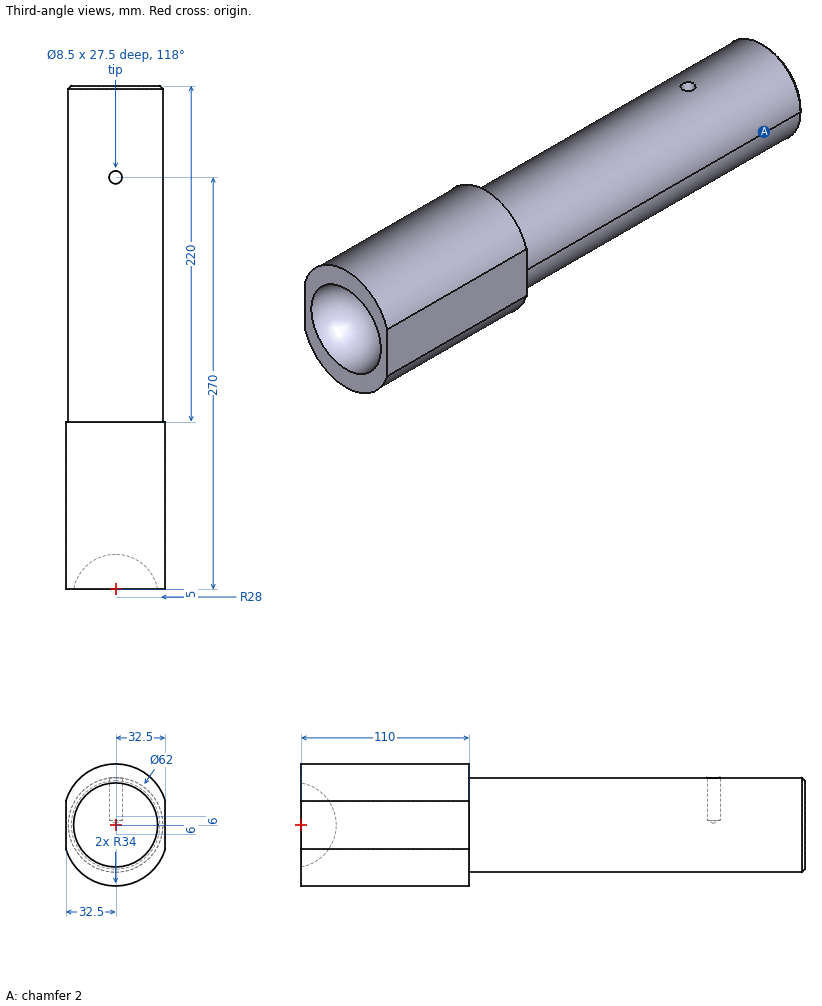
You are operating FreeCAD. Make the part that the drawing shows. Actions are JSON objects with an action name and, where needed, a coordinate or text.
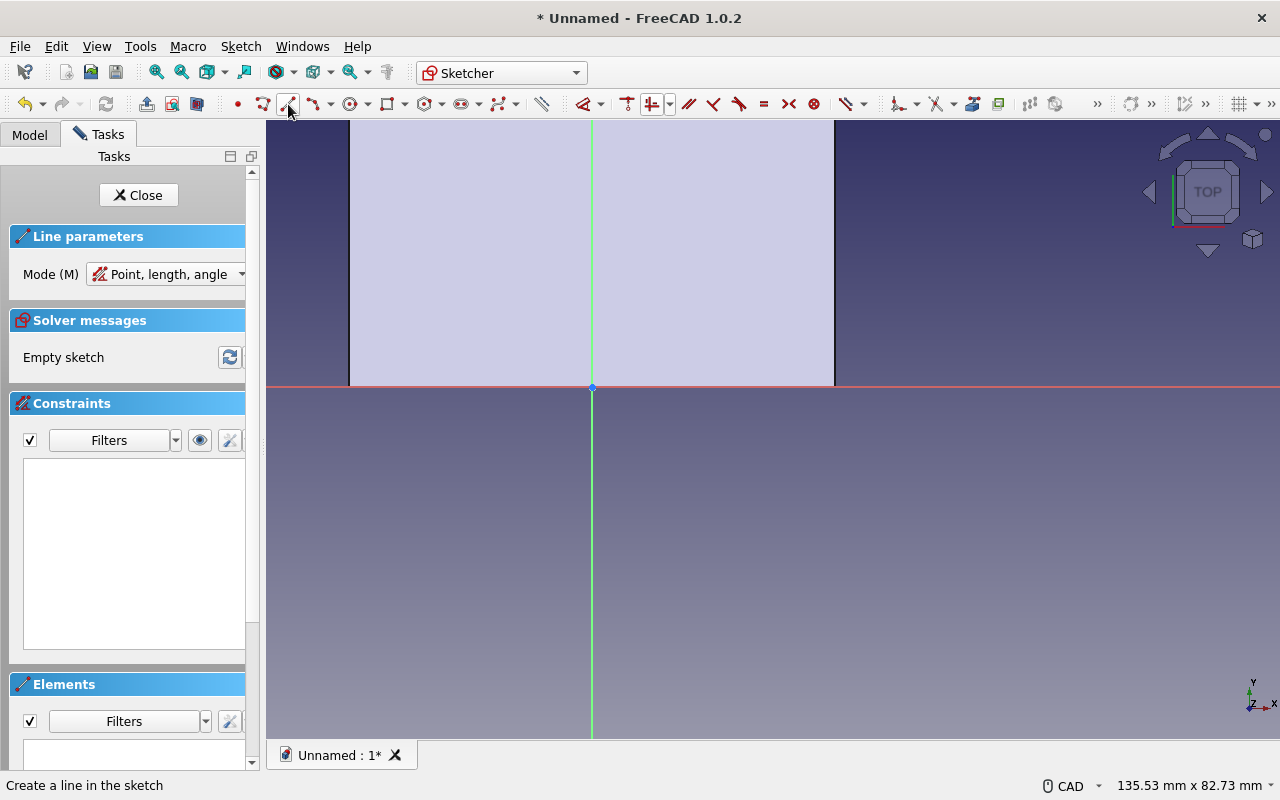
{"action": "left_click", "coordinate": [592, 215]}
{"action": "left_click", "coordinate": [601, 634]}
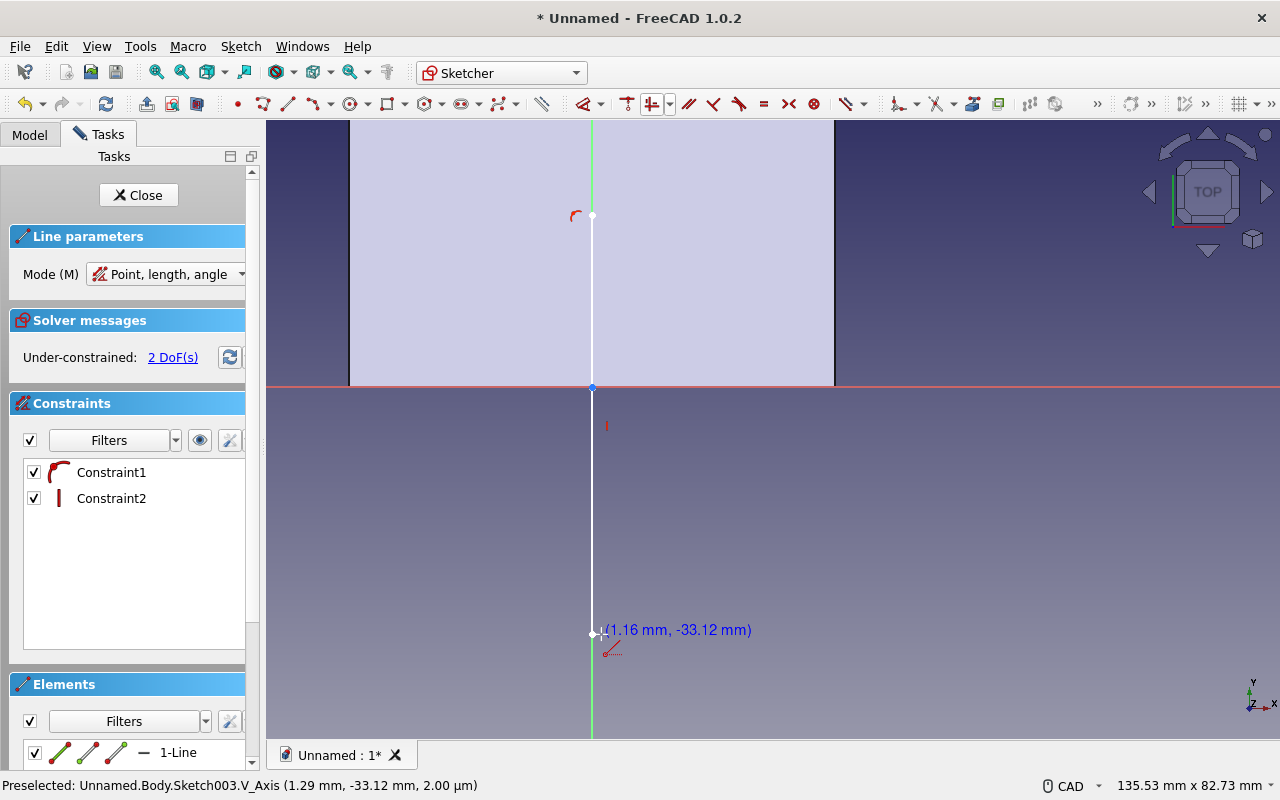
{"action": "key", "text": "g 3 a"}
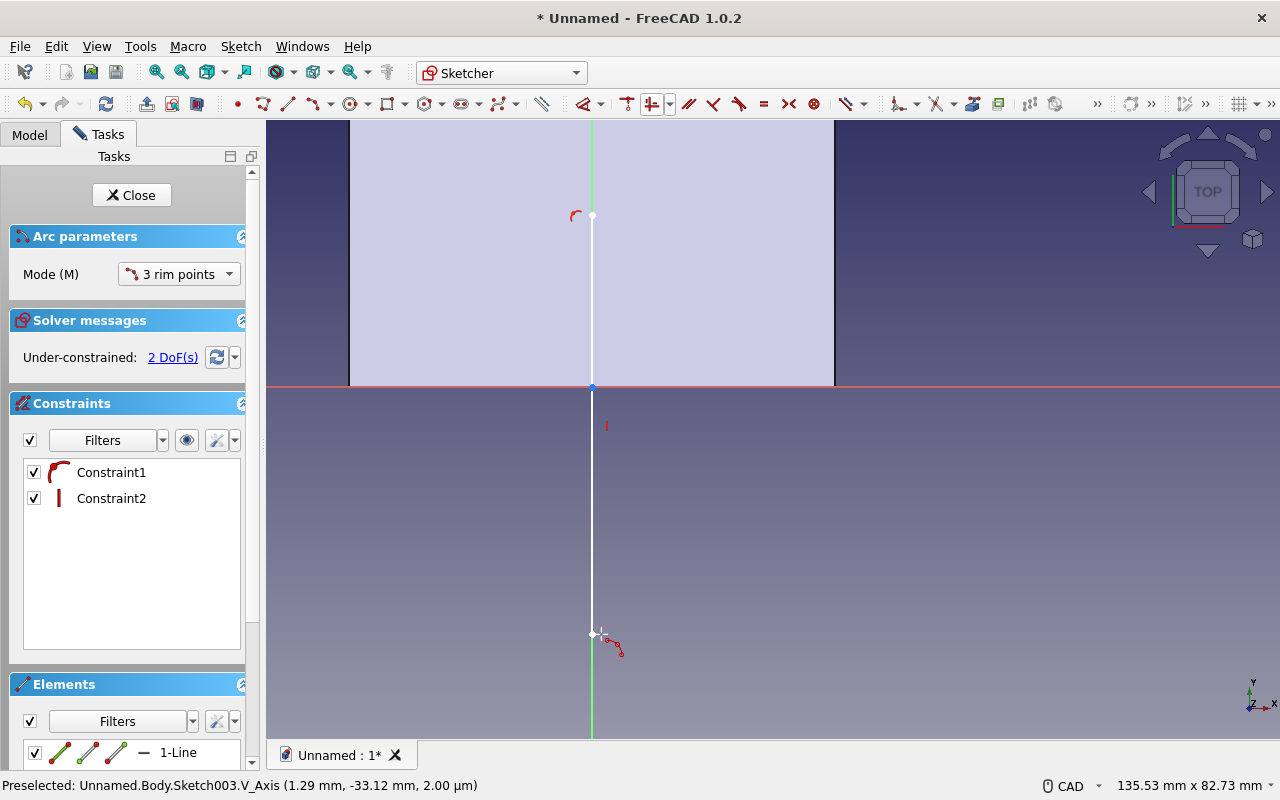
{"action": "left_click", "coordinate": [592, 635]}
{"action": "left_click", "coordinate": [592, 216]}
{"action": "left_click", "coordinate": [802, 425]}
{"action": "key", "text": "Escape"}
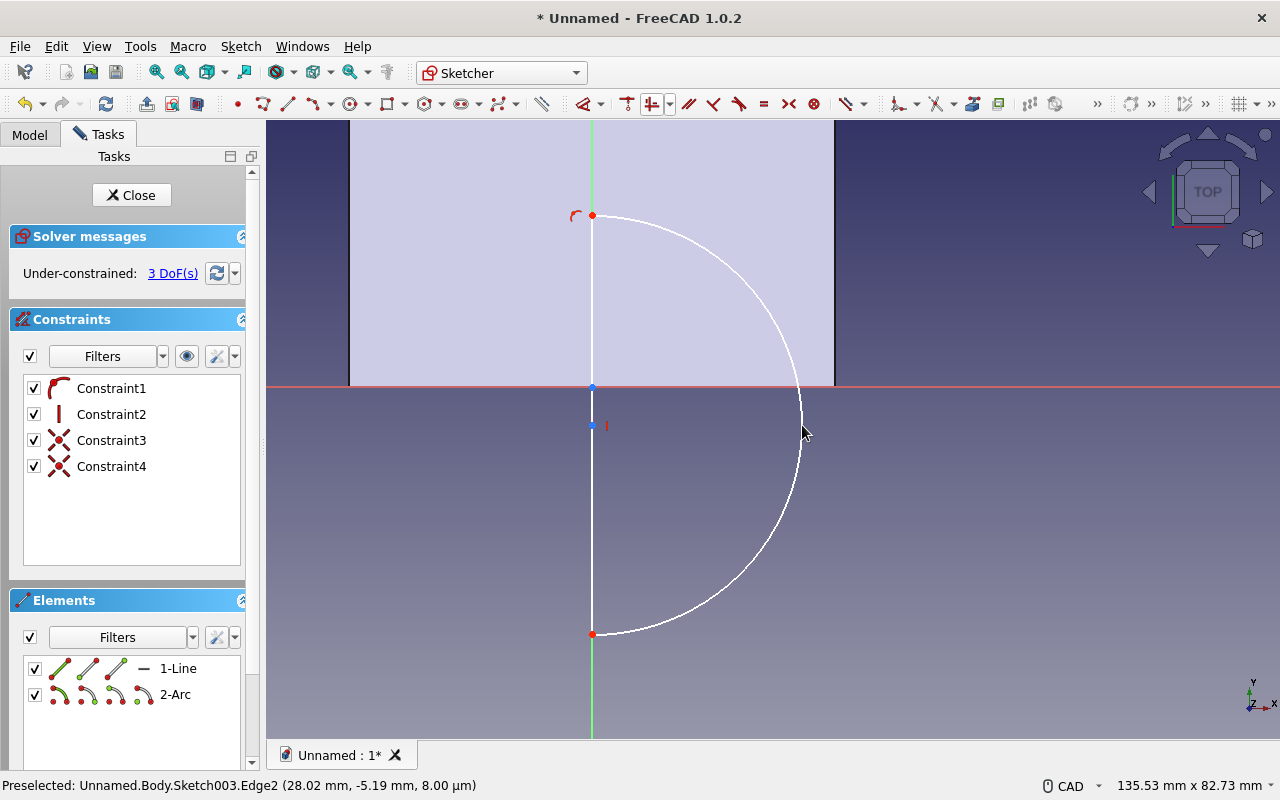
{"action": "left_click", "coordinate": [593, 425]}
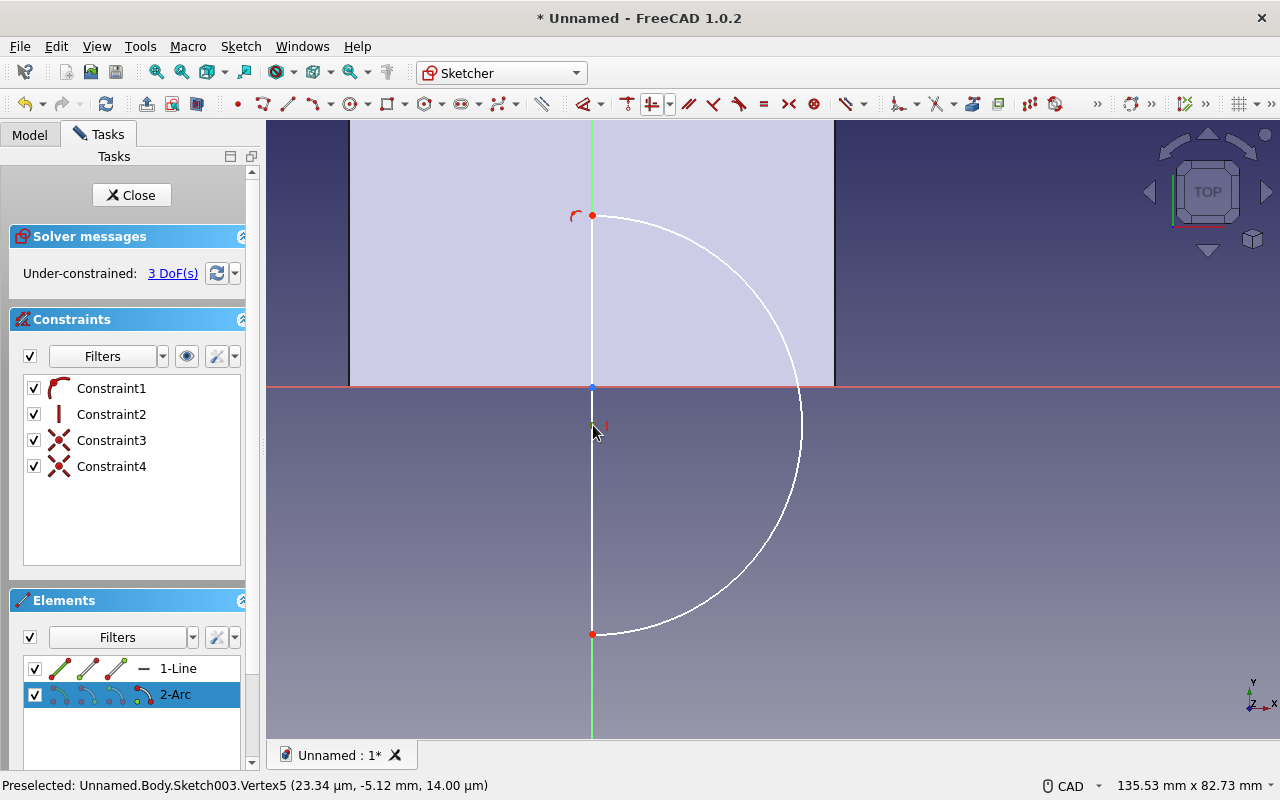
{"action": "left_click", "coordinate": [592, 671]}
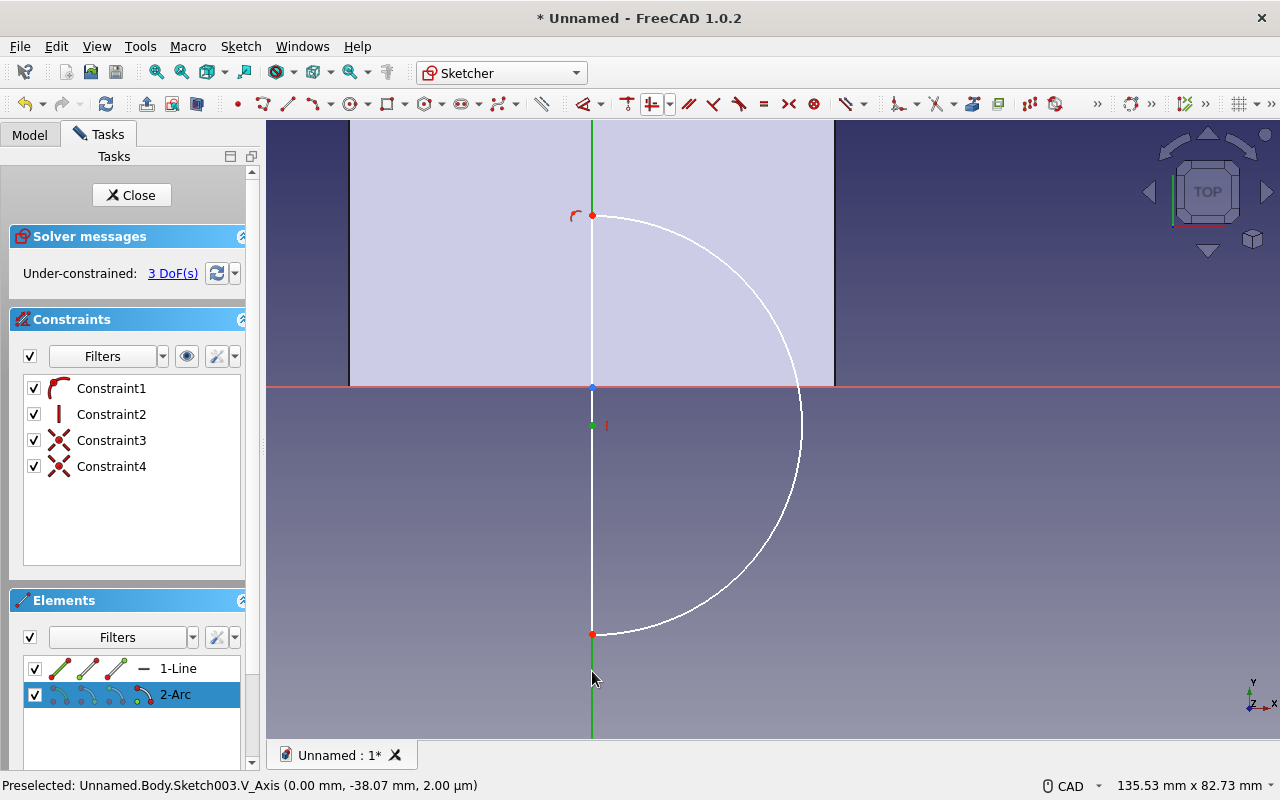
{"action": "left_click", "coordinate": [627, 104]}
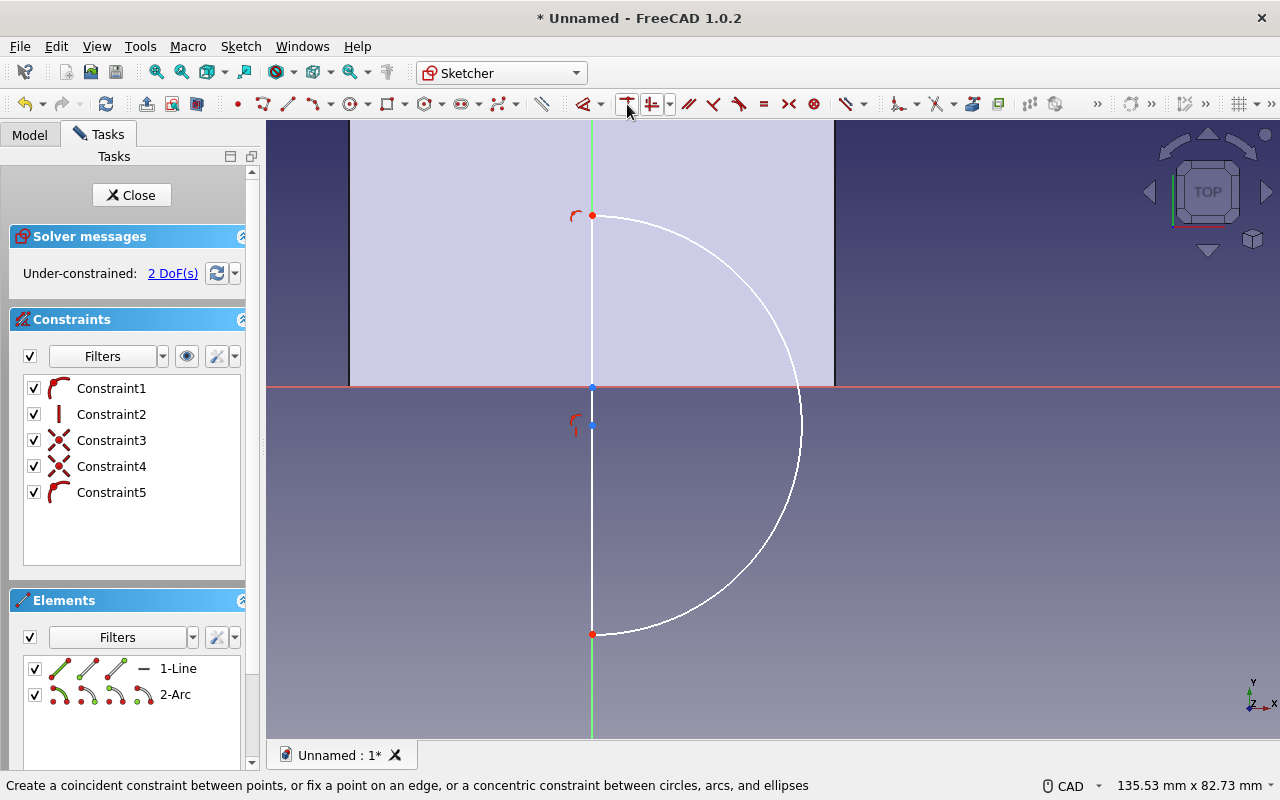
{"action": "left_click", "coordinate": [582, 104]}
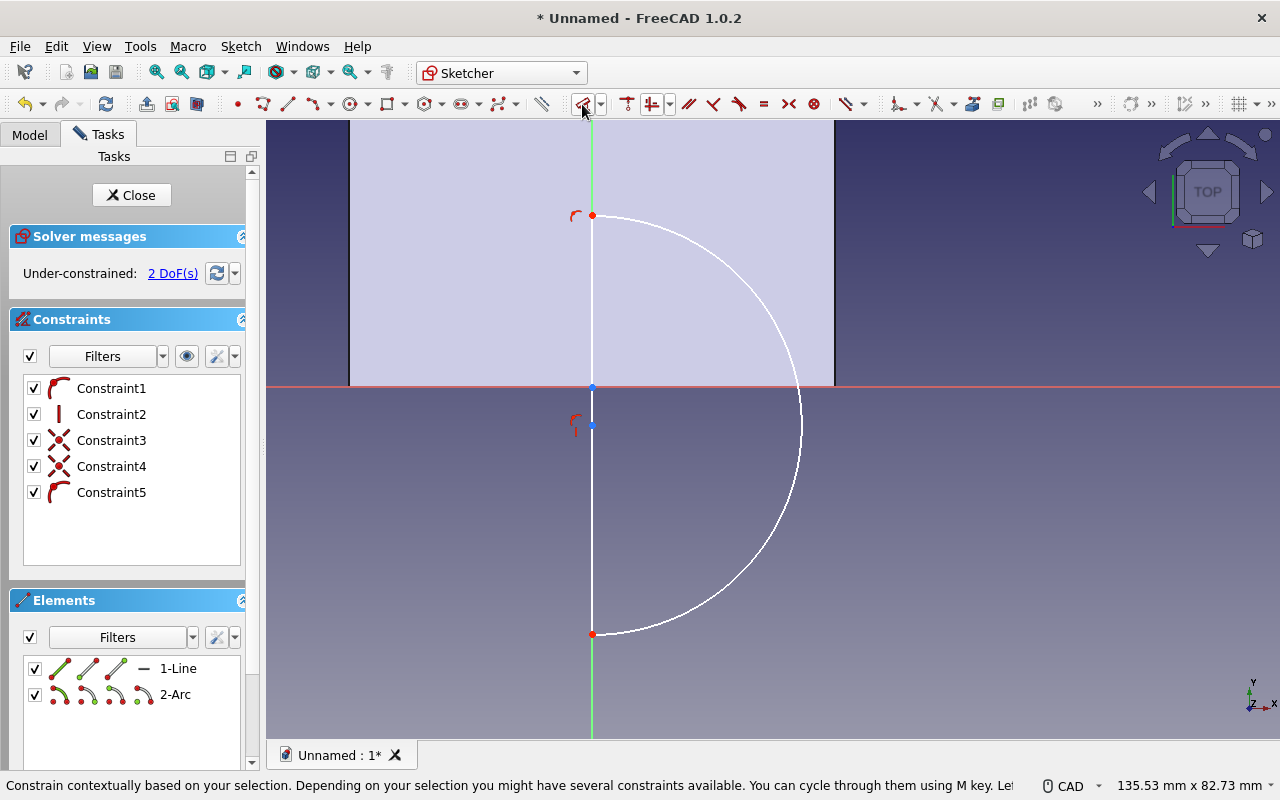
{"action": "left_click", "coordinate": [762, 549]}
{"action": "left_click", "coordinate": [788, 568]}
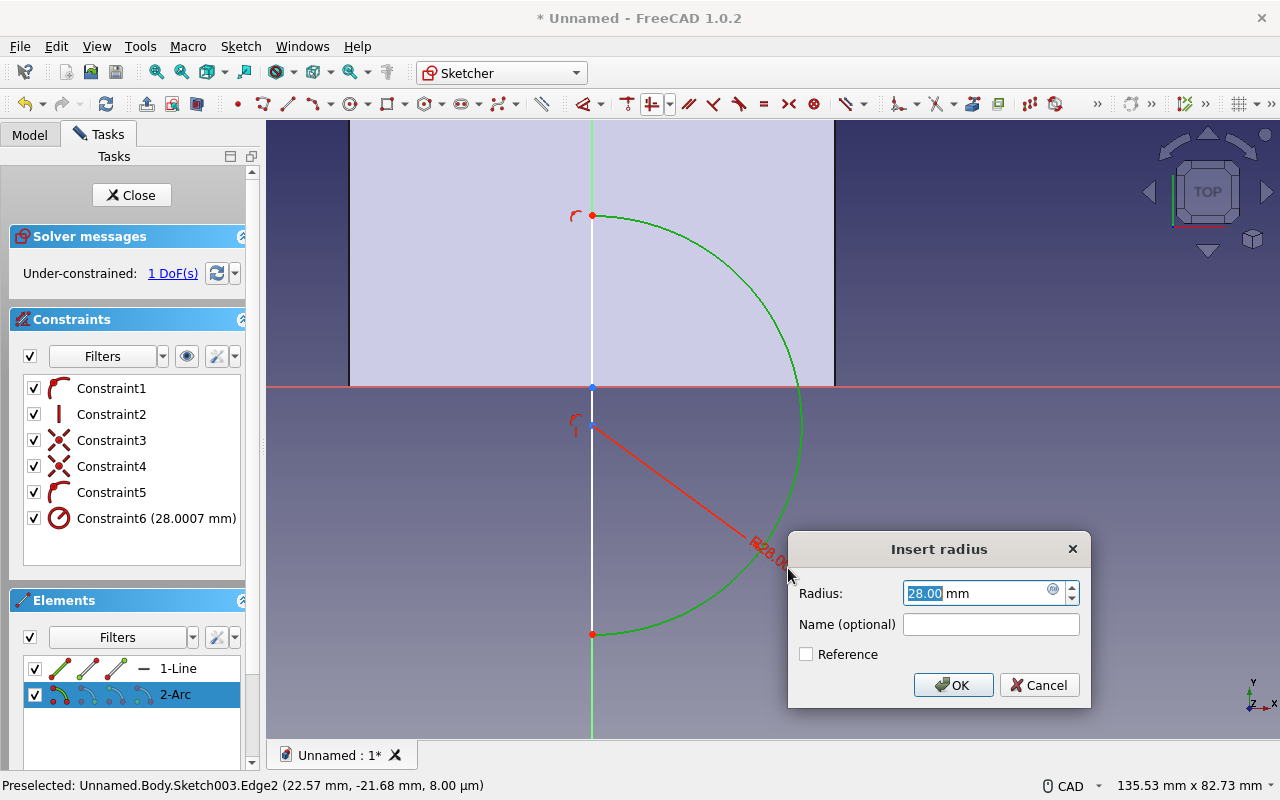
{"action": "type", "text": "28"}
{"action": "key", "text": "Return"}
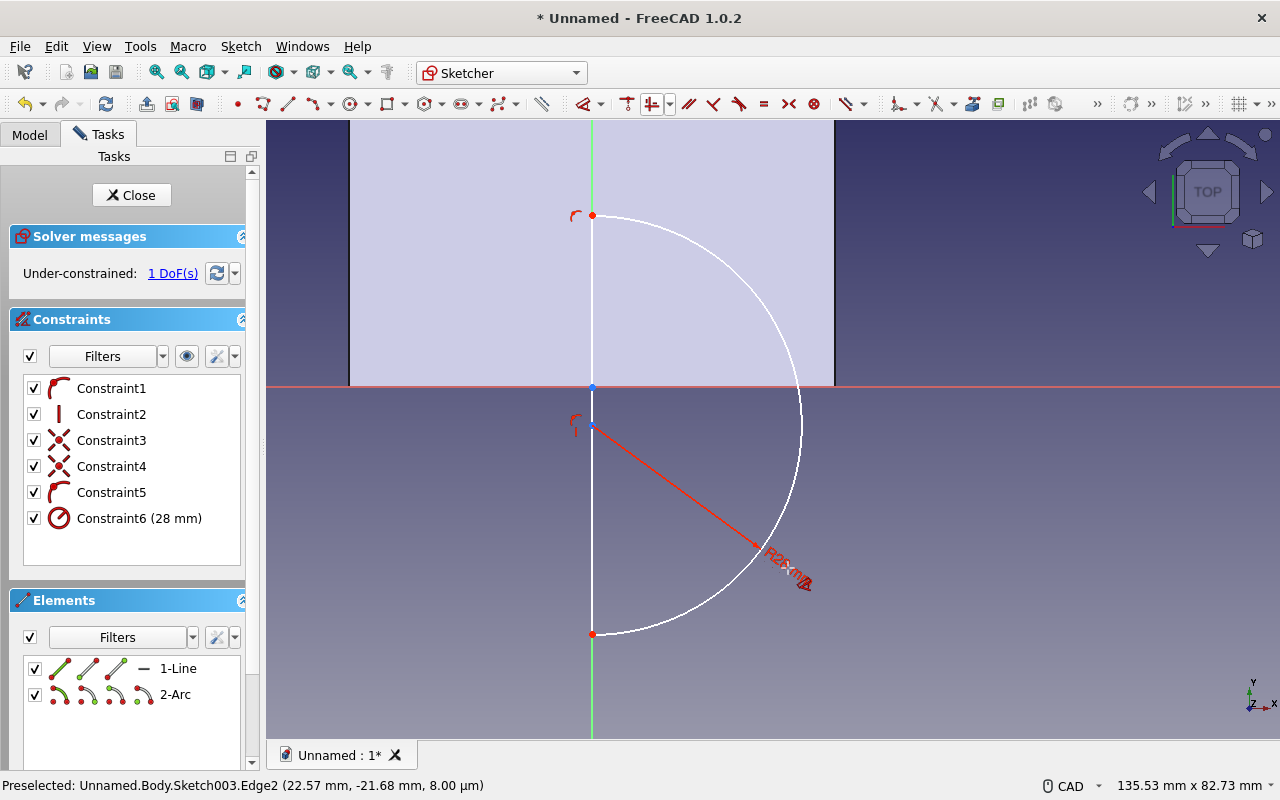
{"action": "left_click", "coordinate": [592, 425]}
{"action": "left_click", "coordinate": [558, 406]}